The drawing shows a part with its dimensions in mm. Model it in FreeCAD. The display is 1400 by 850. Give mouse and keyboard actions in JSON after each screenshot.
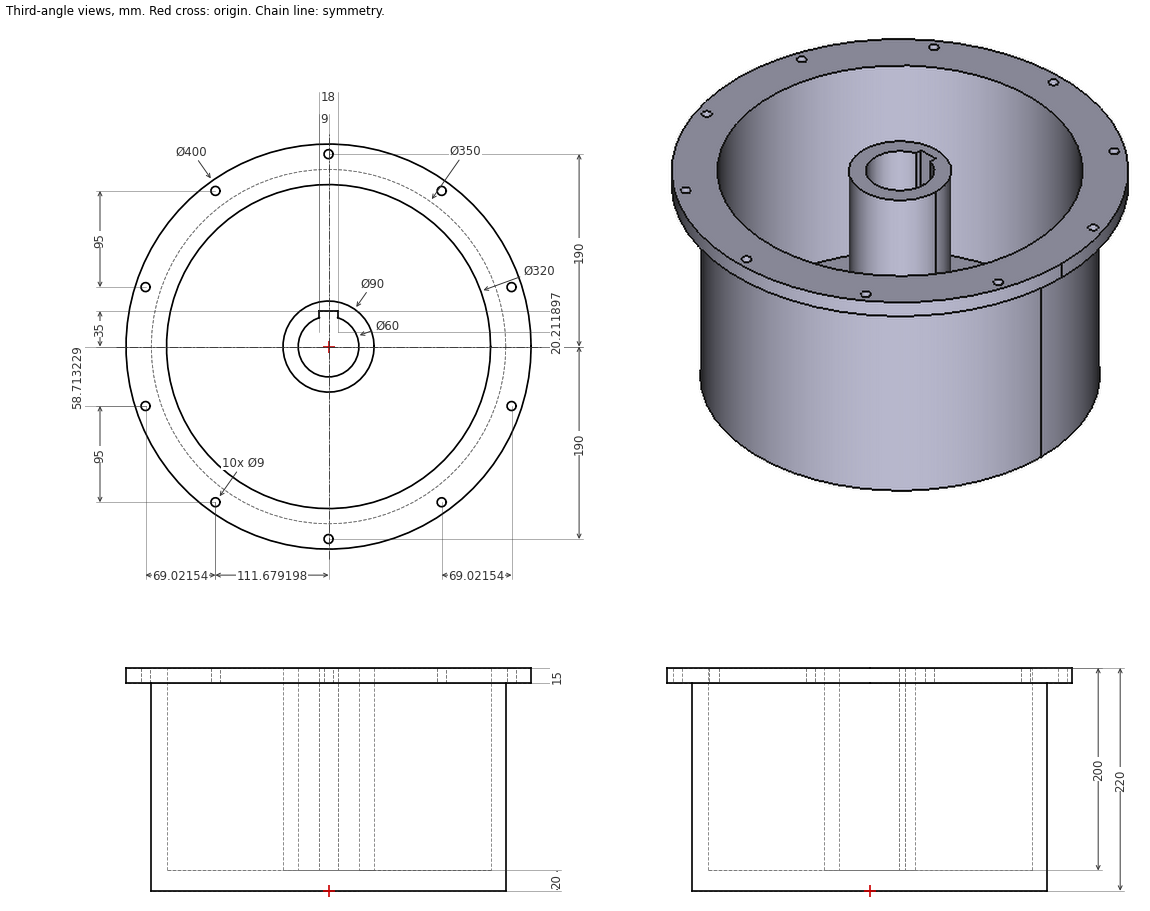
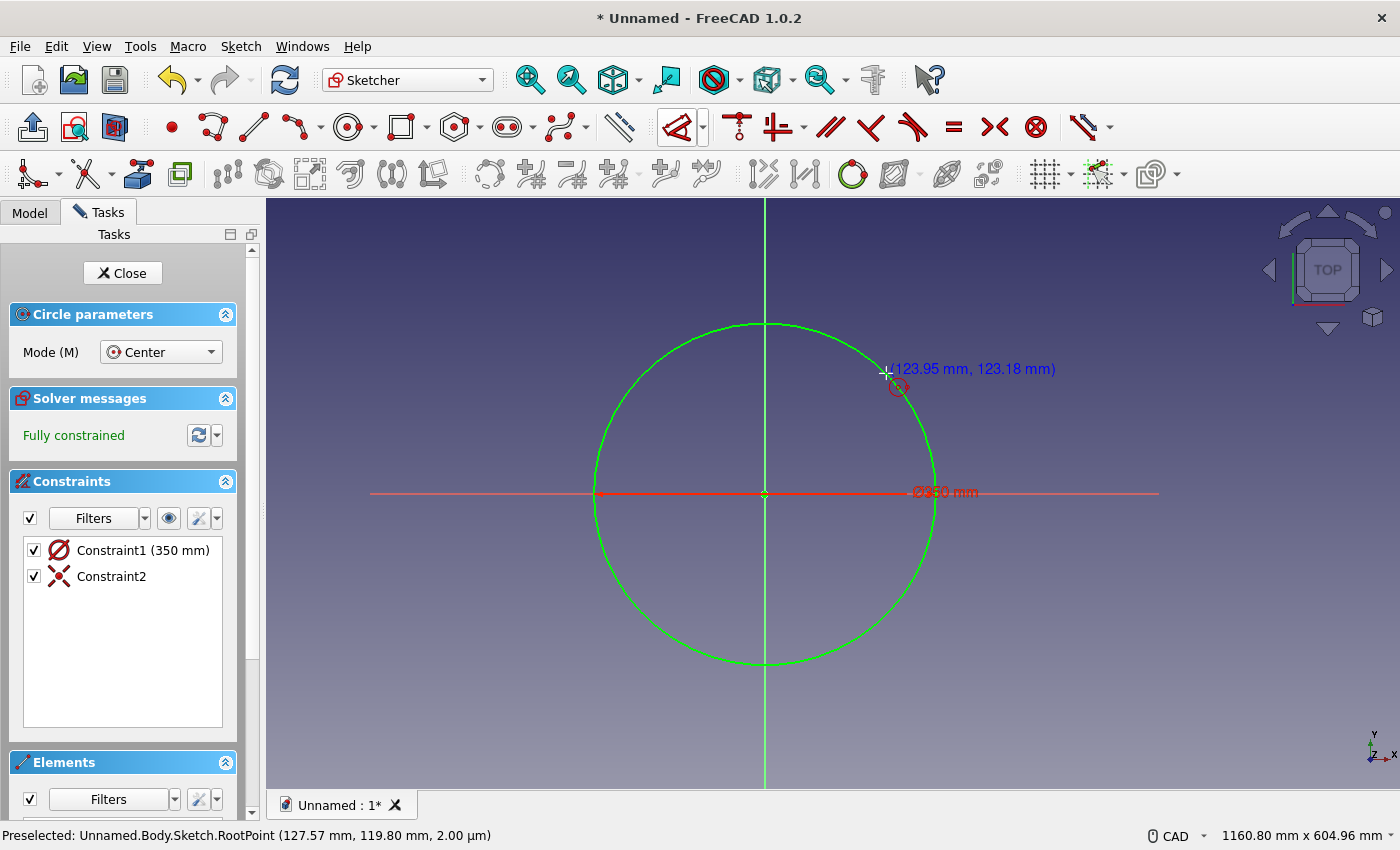
{"action": "left_click", "coordinate": [765, 494]}
{"action": "mouse_move", "coordinate": [786, 474]}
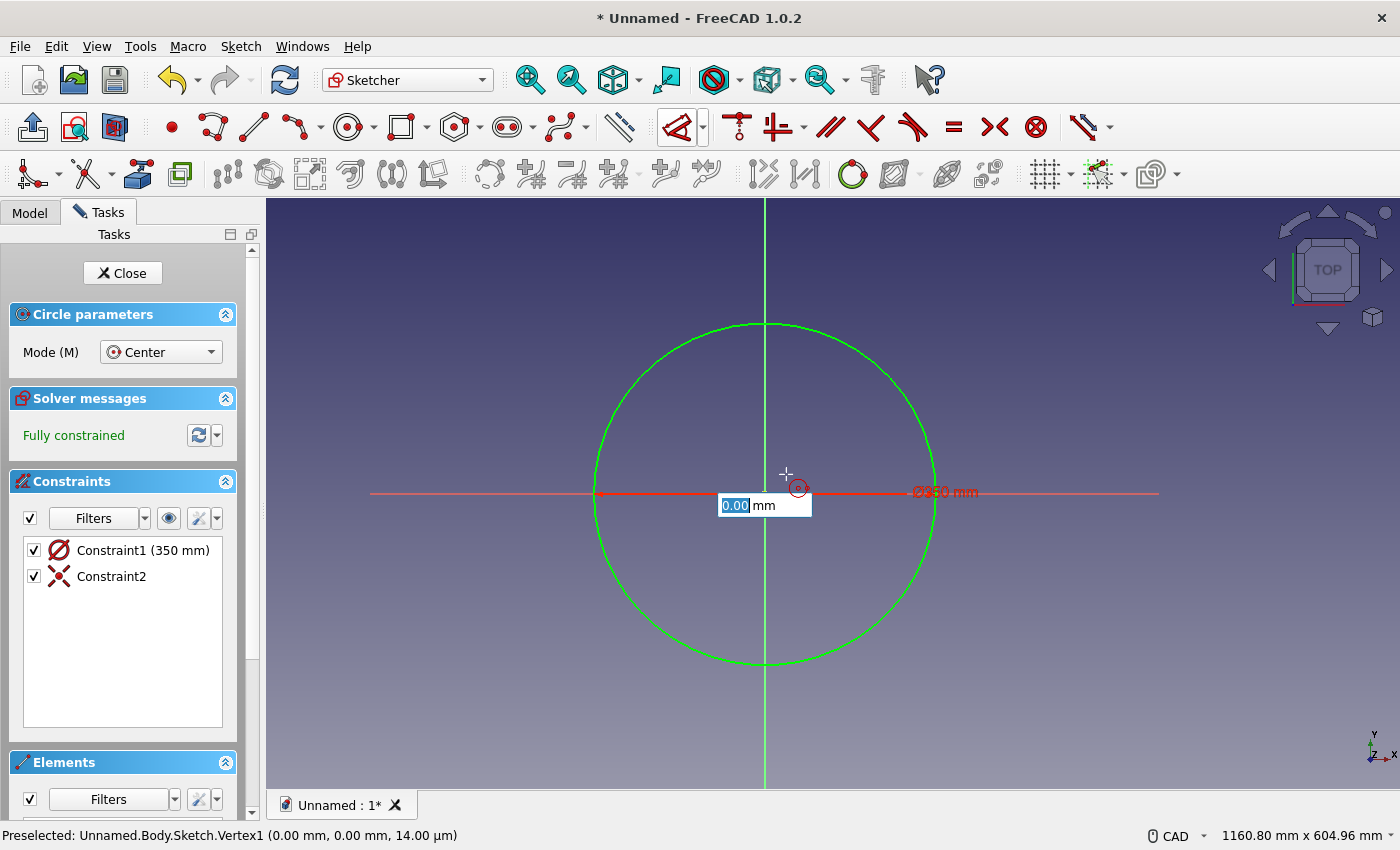
{"action": "type", "text": "60"}
{"action": "key", "text": "Return"}
{"action": "key", "text": "Escape"}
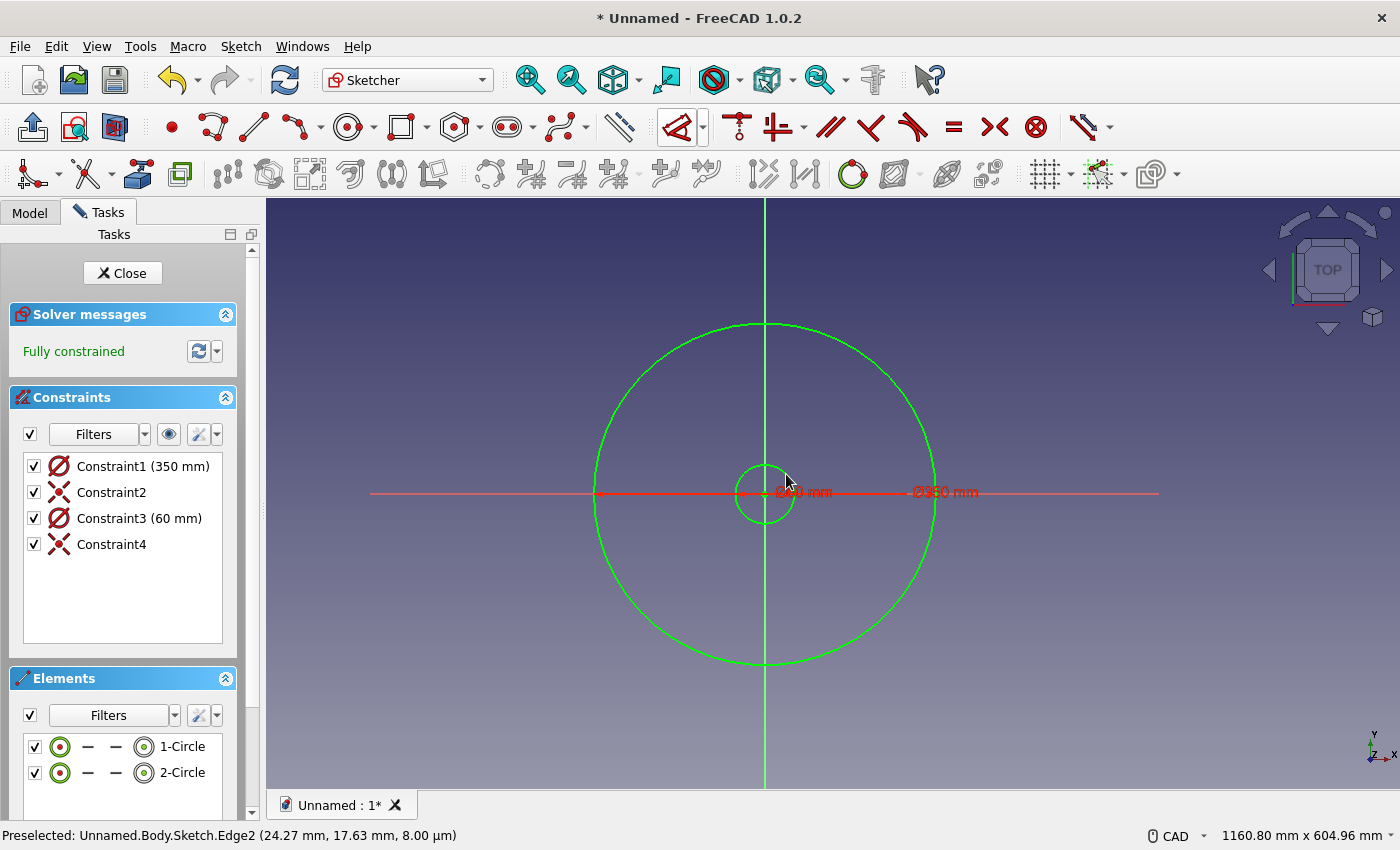
{"action": "left_click", "coordinate": [123, 273]}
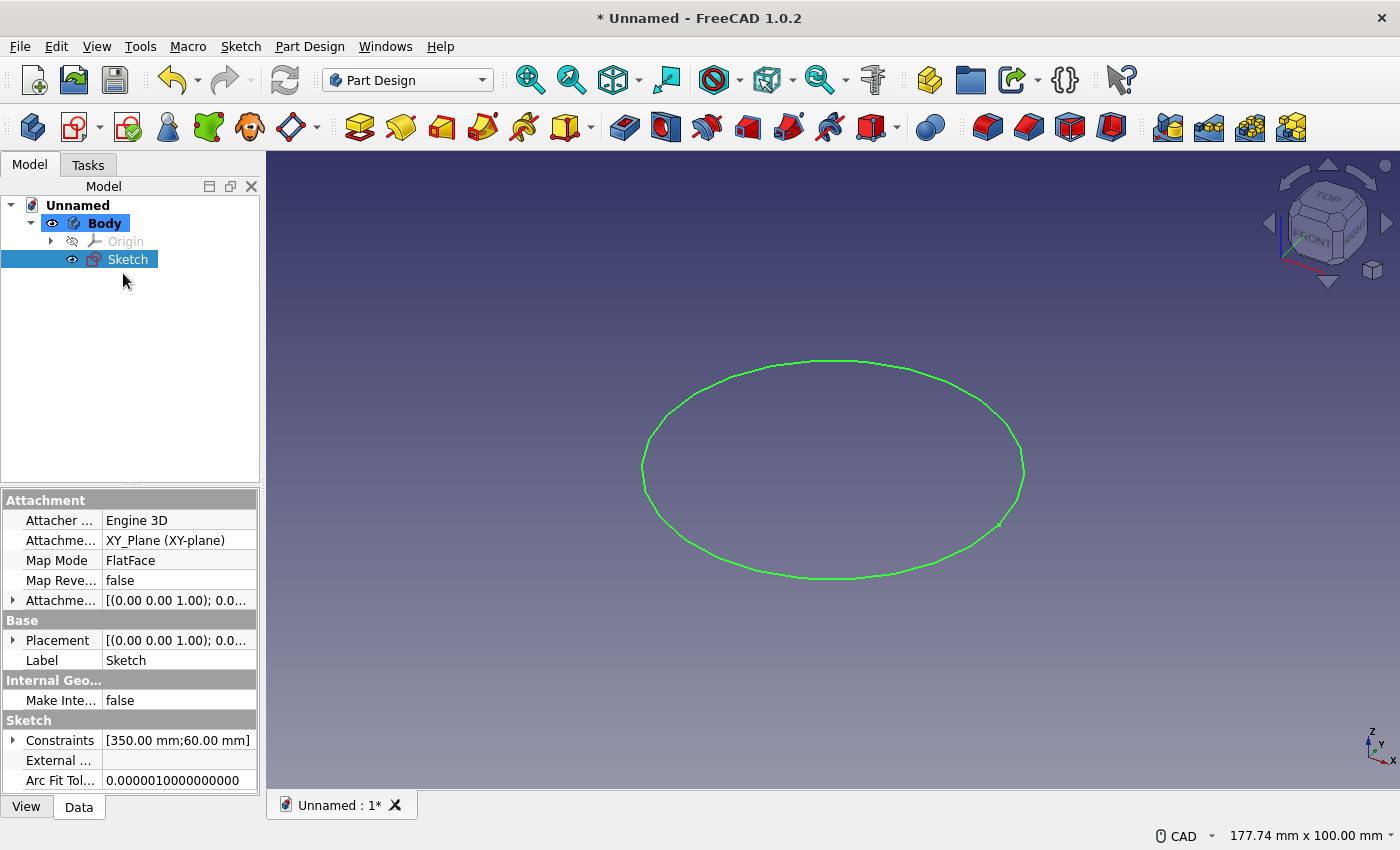
{"action": "left_click", "coordinate": [360, 128]}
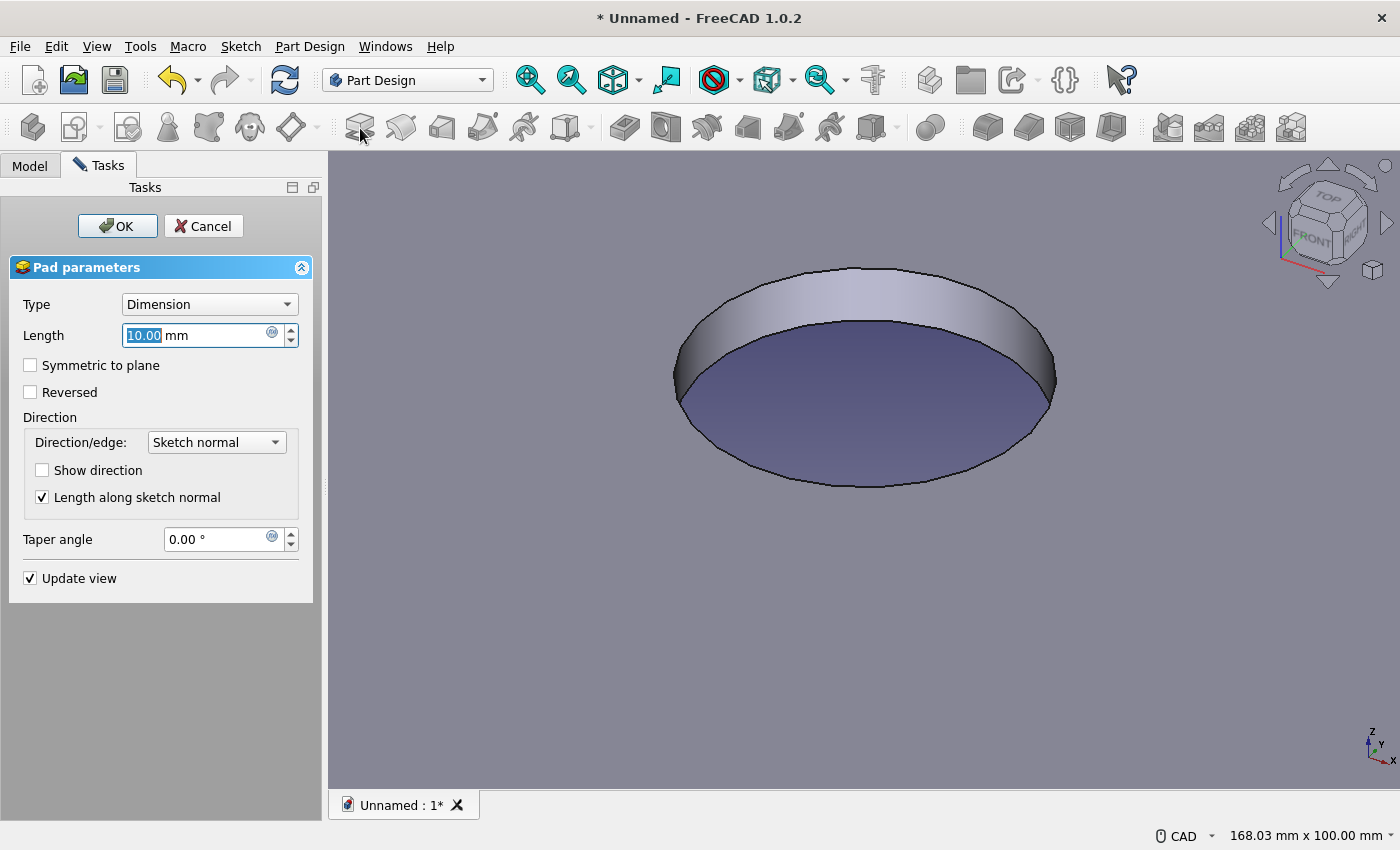
{"action": "type", "text": "220"}
{"action": "key", "text": "Tab"}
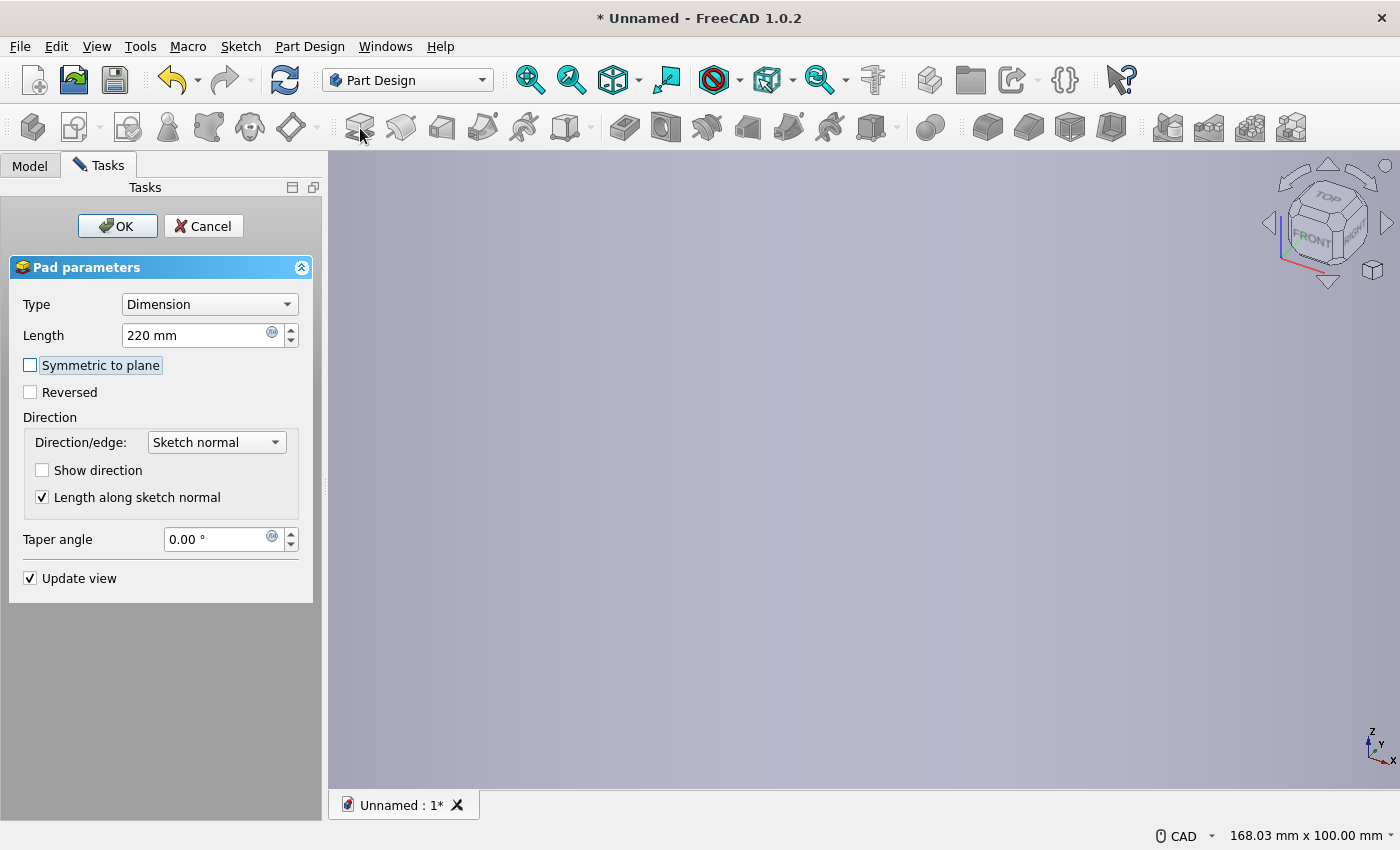
{"action": "left_click", "coordinate": [118, 226]}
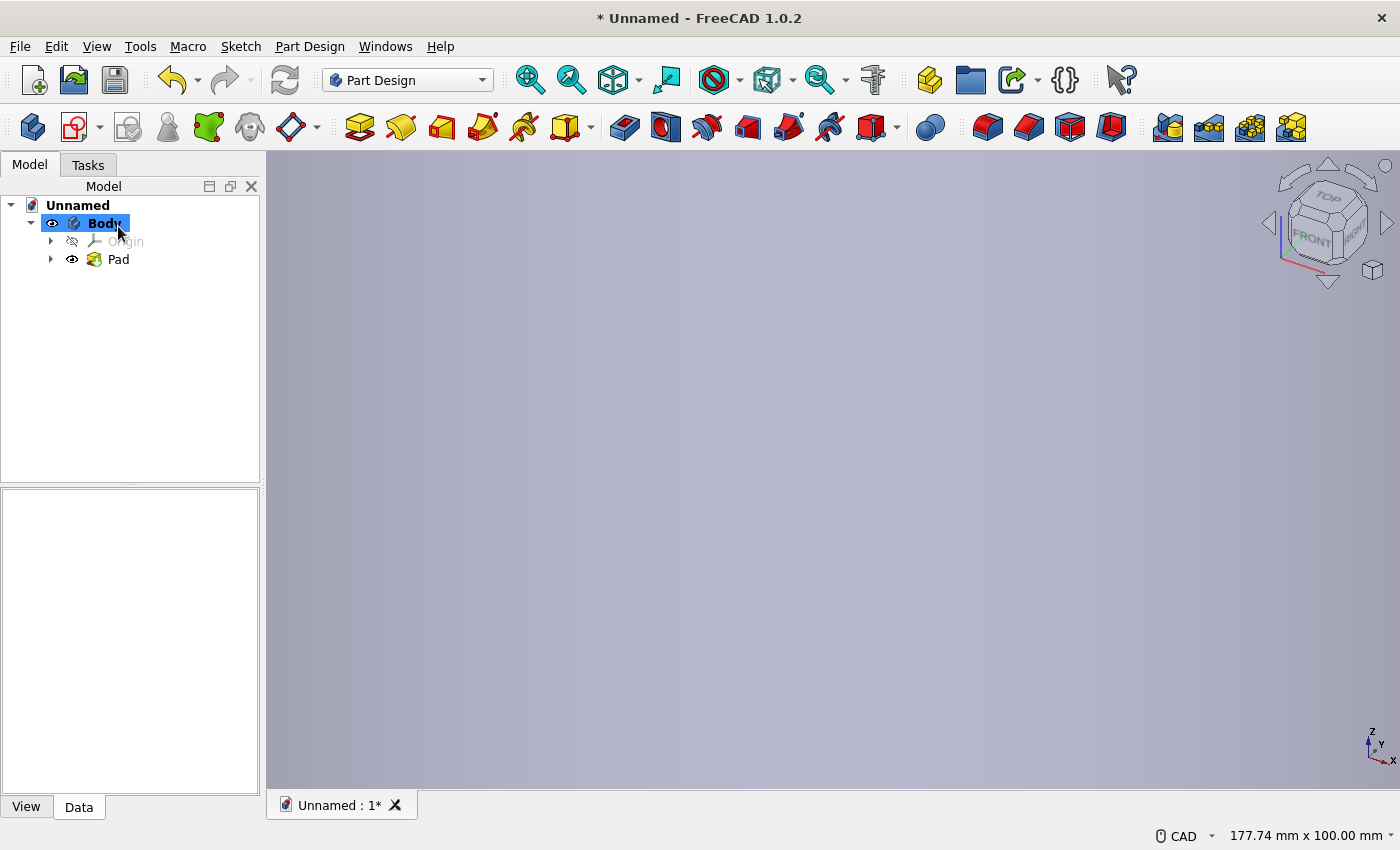
{"action": "left_click", "coordinate": [531, 80]}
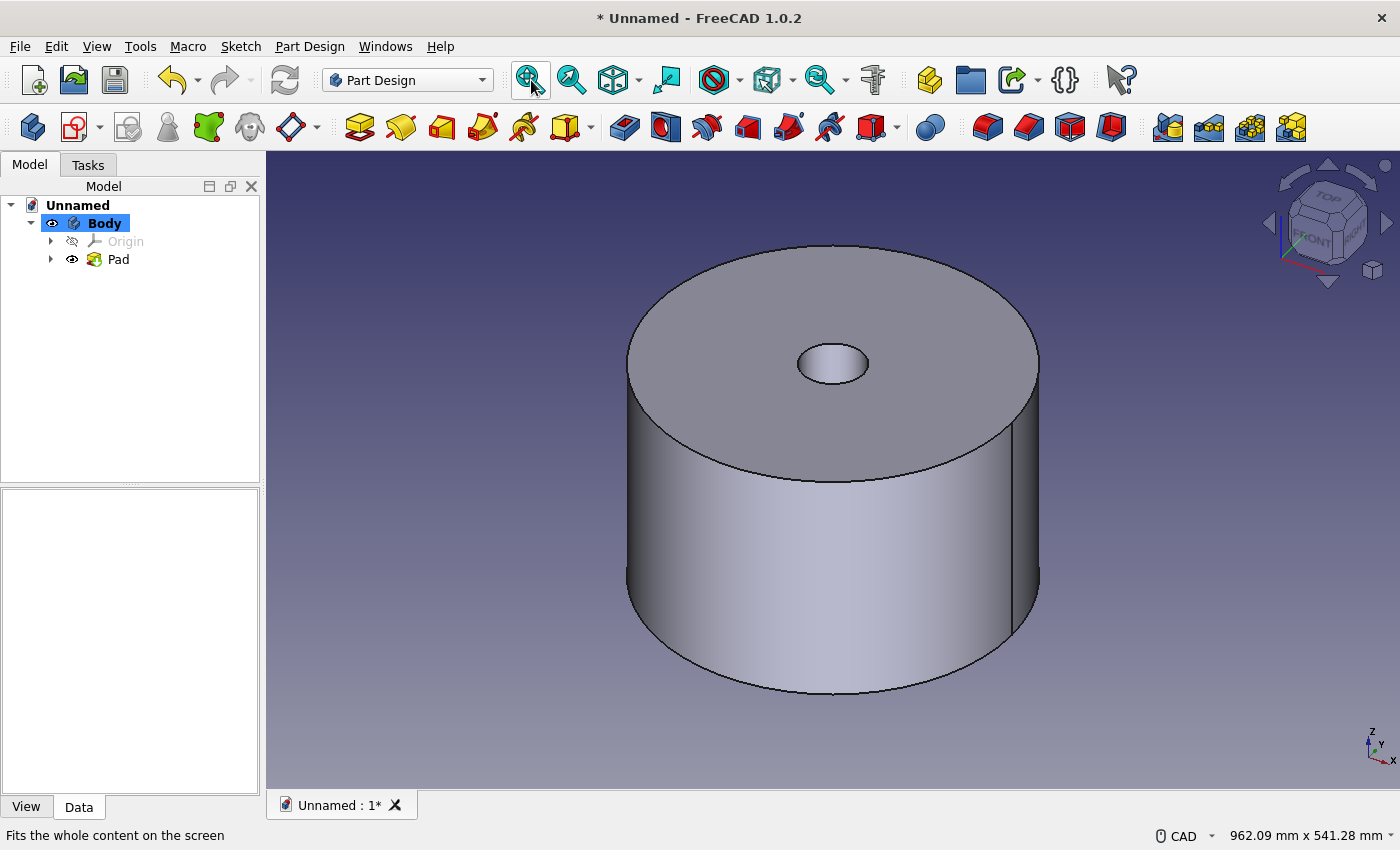
{"action": "left_click", "coordinate": [51, 241]}